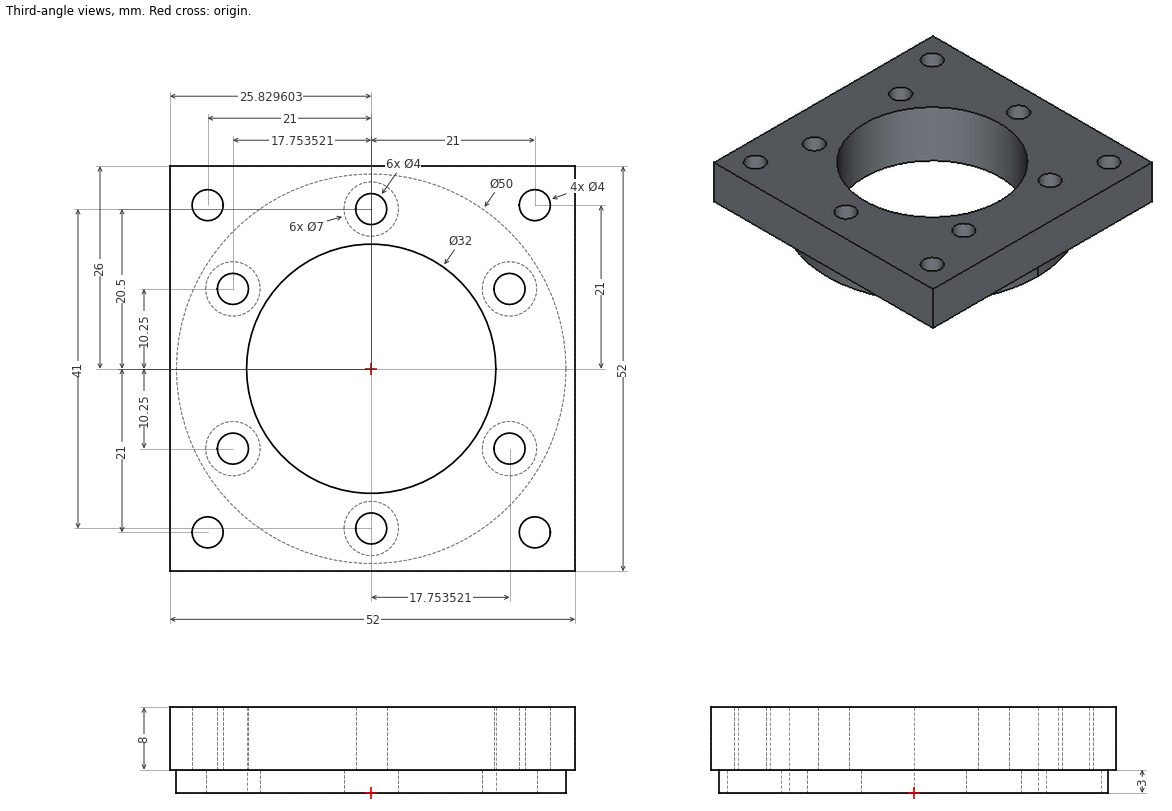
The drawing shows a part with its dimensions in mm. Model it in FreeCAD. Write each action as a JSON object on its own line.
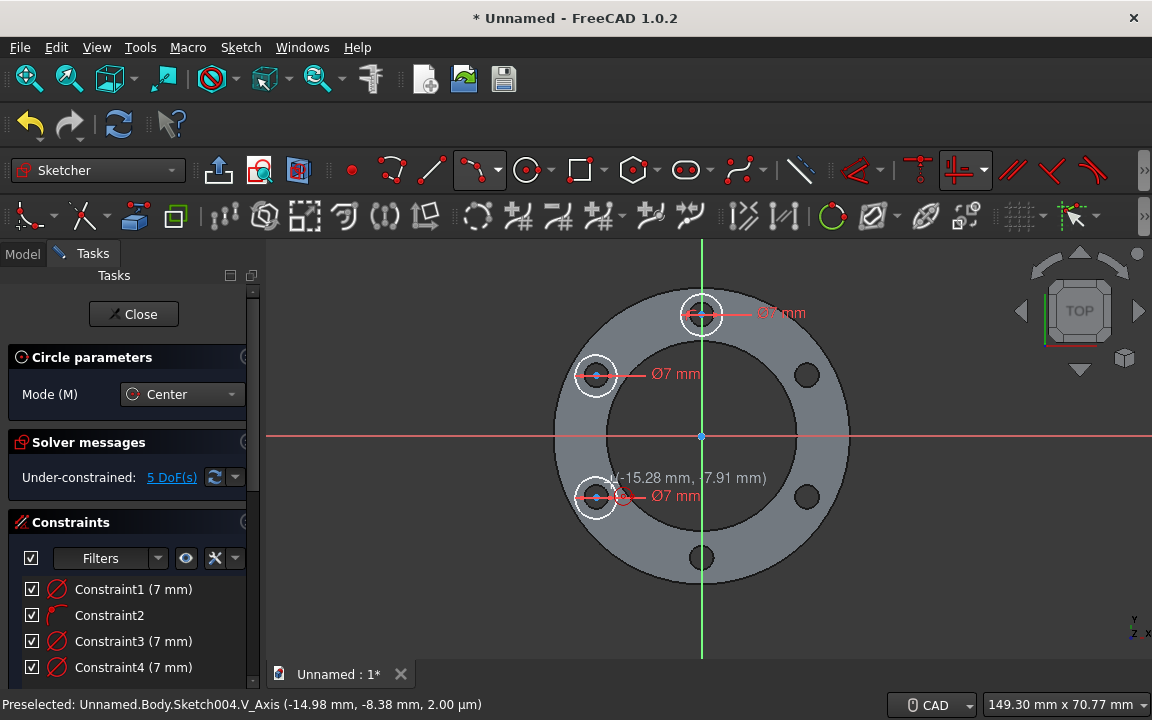
{"action": "left_click", "coordinate": [702, 558]}
{"action": "mouse_move", "coordinate": [716, 543]}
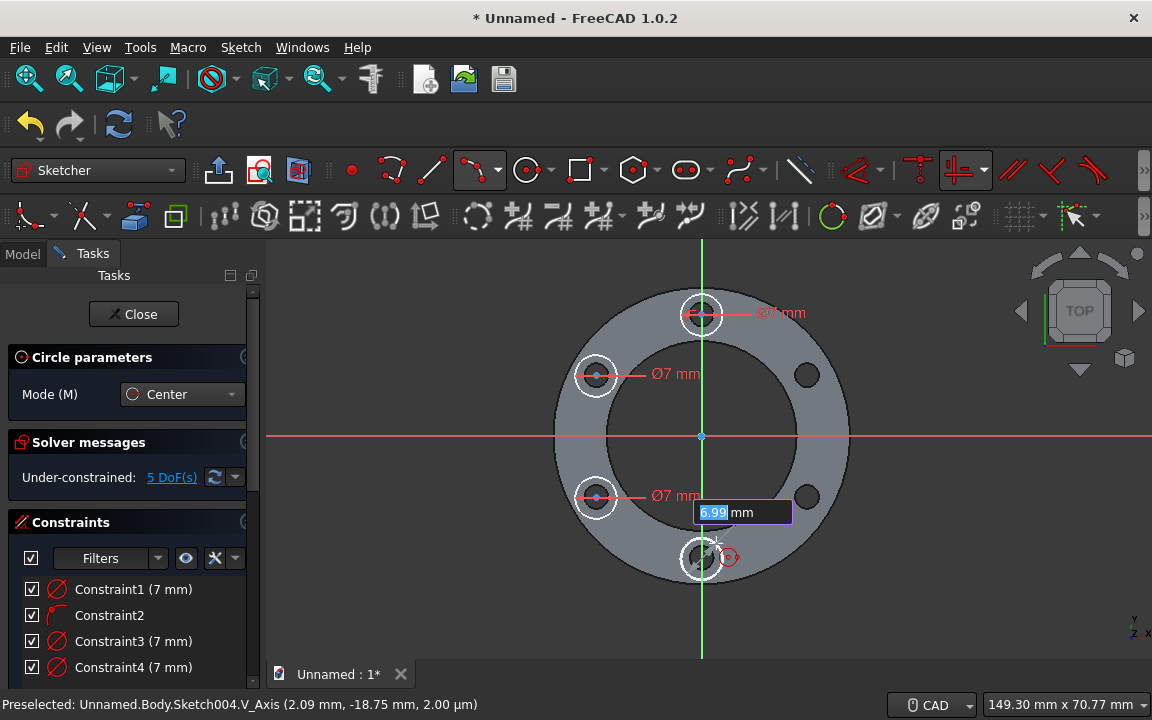
{"action": "type", "text": "7"}
{"action": "key", "text": "Return"}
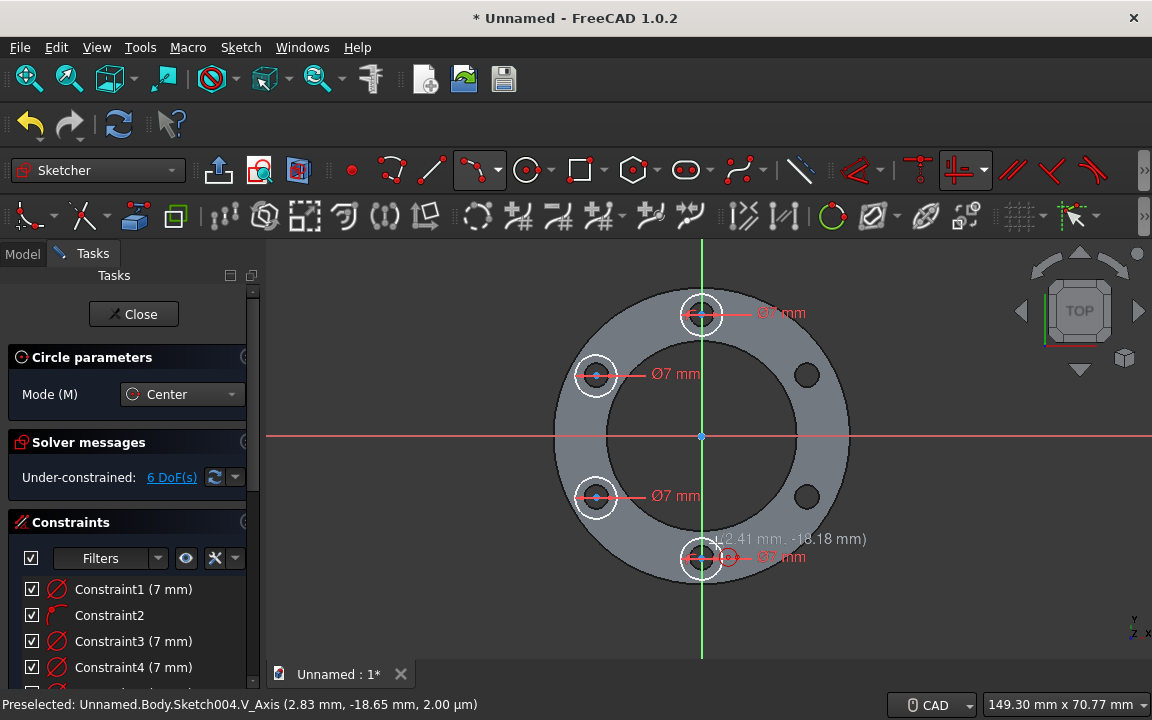
{"action": "left_click", "coordinate": [807, 497]}
{"action": "mouse_move", "coordinate": [822, 482]}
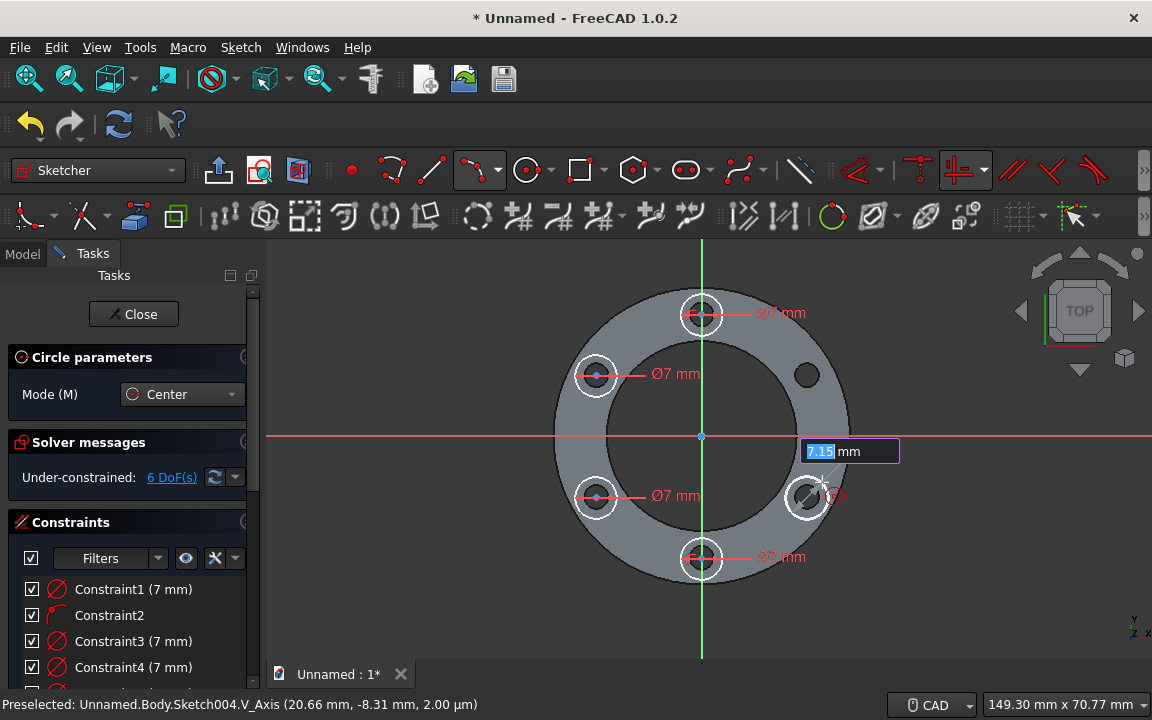
{"action": "type", "text": "7"}
{"action": "key", "text": "Return"}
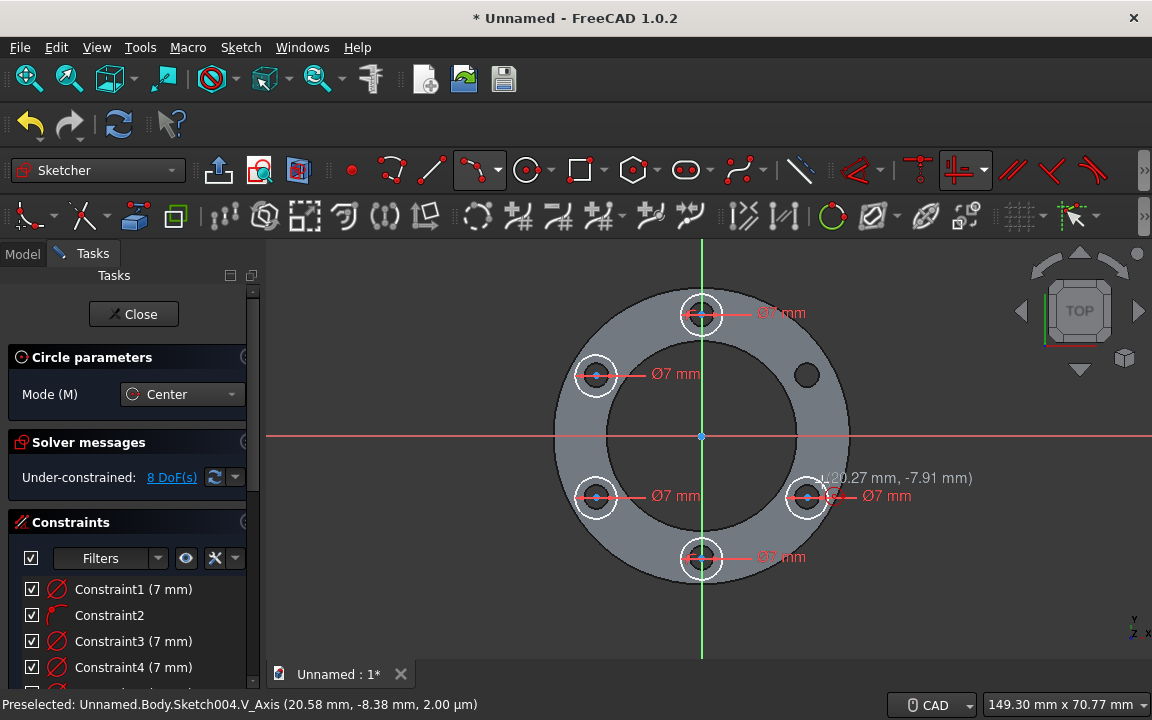
{"action": "left_click", "coordinate": [807, 375]}
{"action": "mouse_move", "coordinate": [822, 361]}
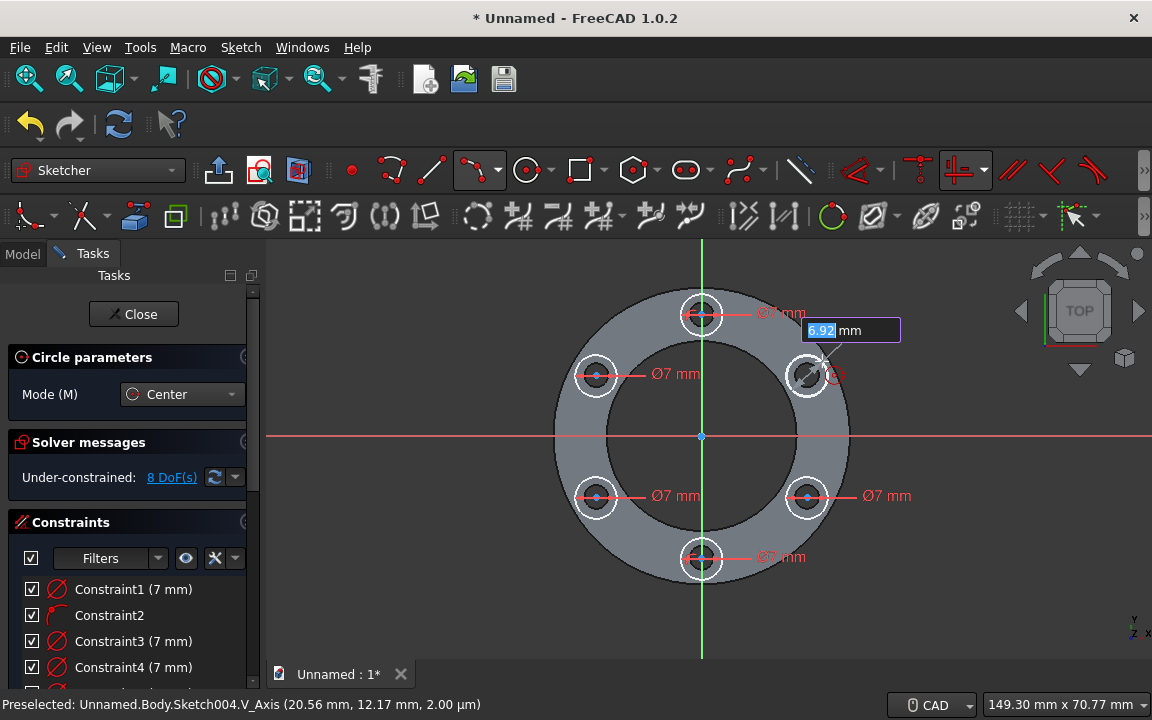
{"action": "type", "text": "7"}
{"action": "key", "text": "Return"}
{"action": "key", "text": "Escape"}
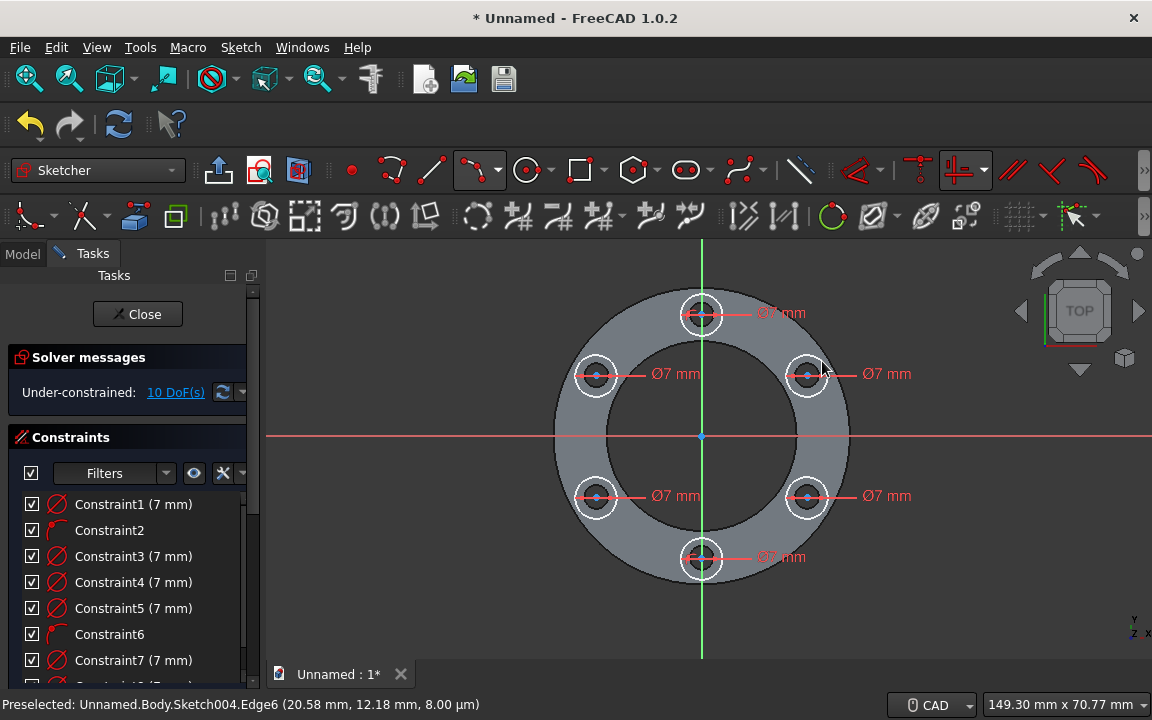
{"action": "left_click", "coordinate": [596, 376]}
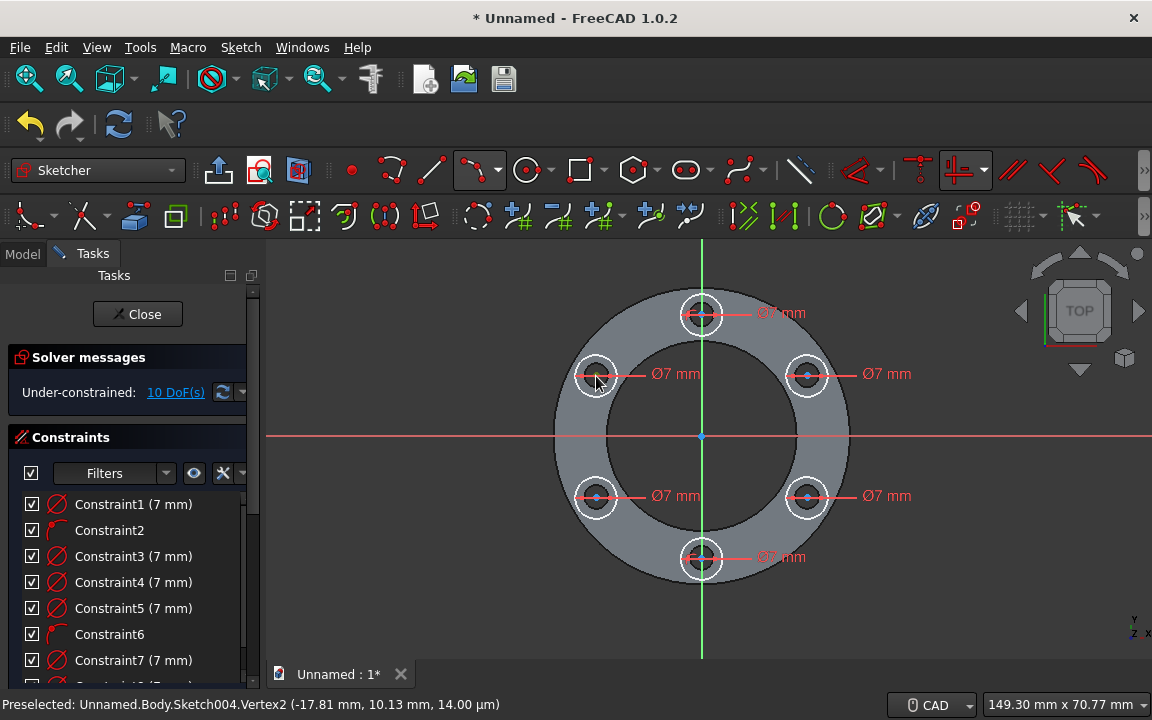
{"action": "left_click", "coordinate": [596, 498]}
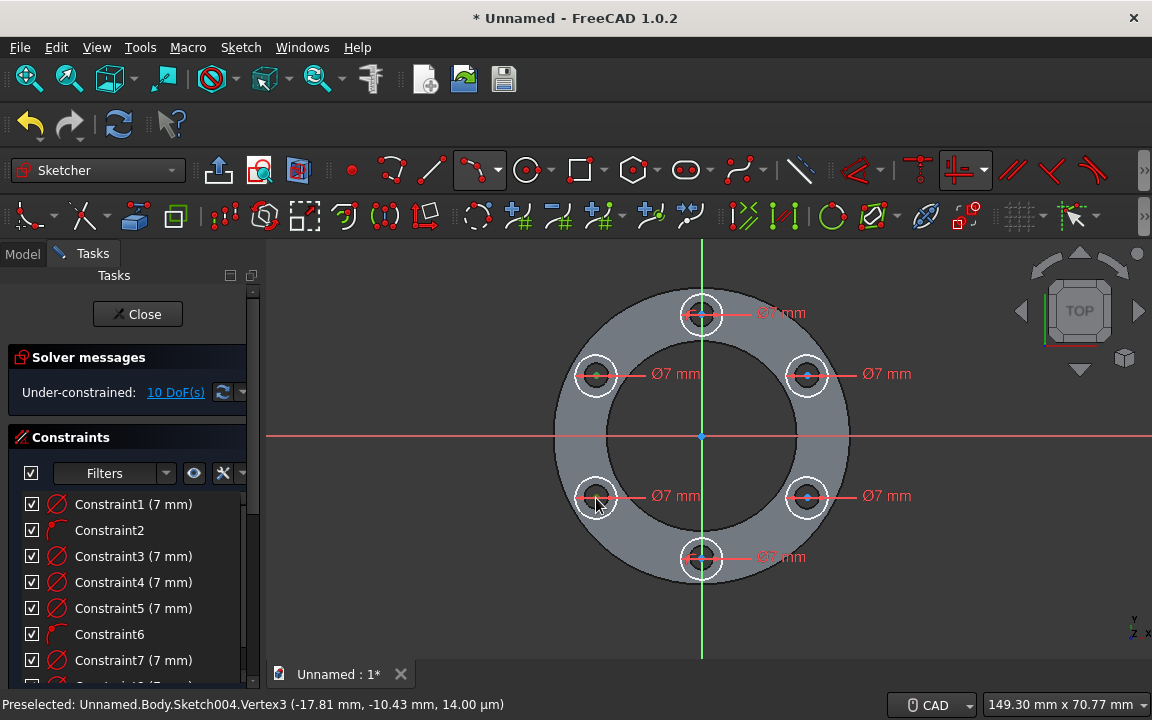
{"action": "key", "text": "v"}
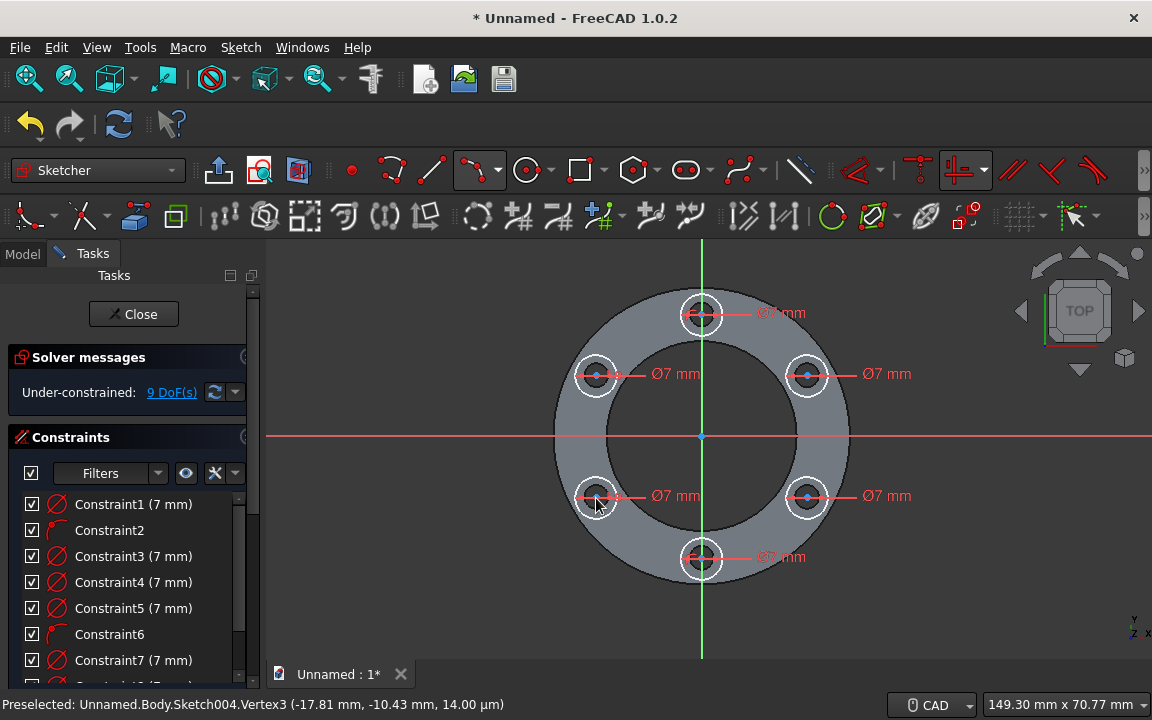
{"action": "left_click", "coordinate": [596, 498]}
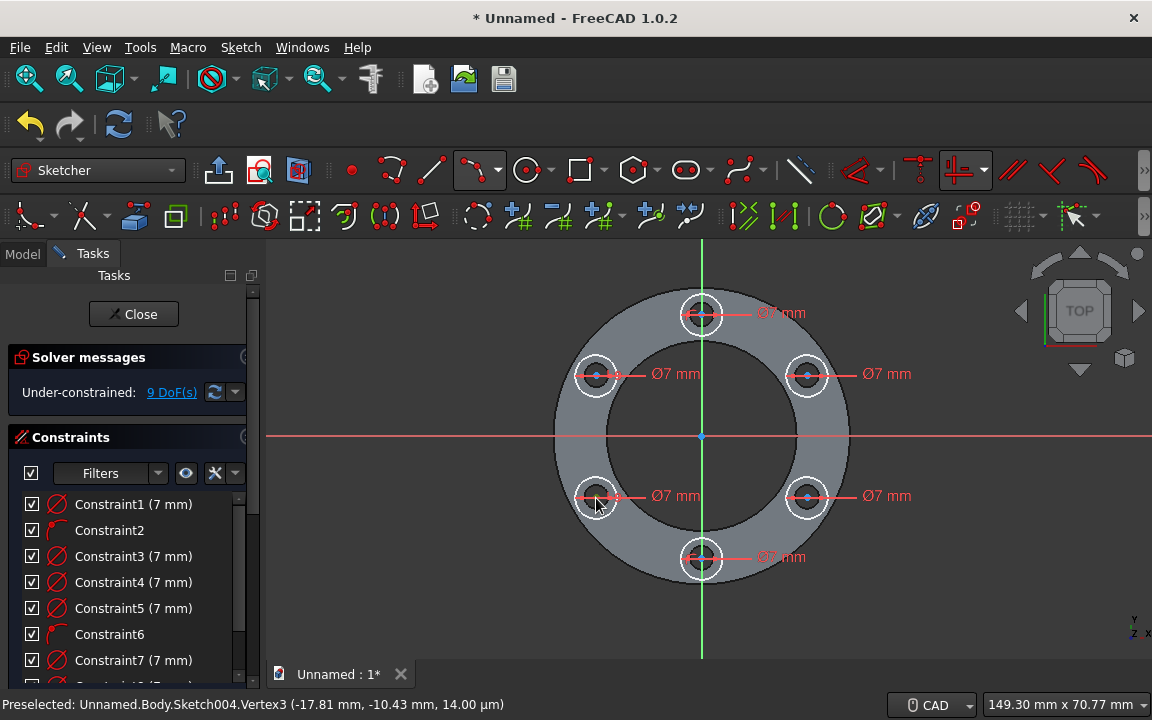
{"action": "left_click", "coordinate": [807, 498]}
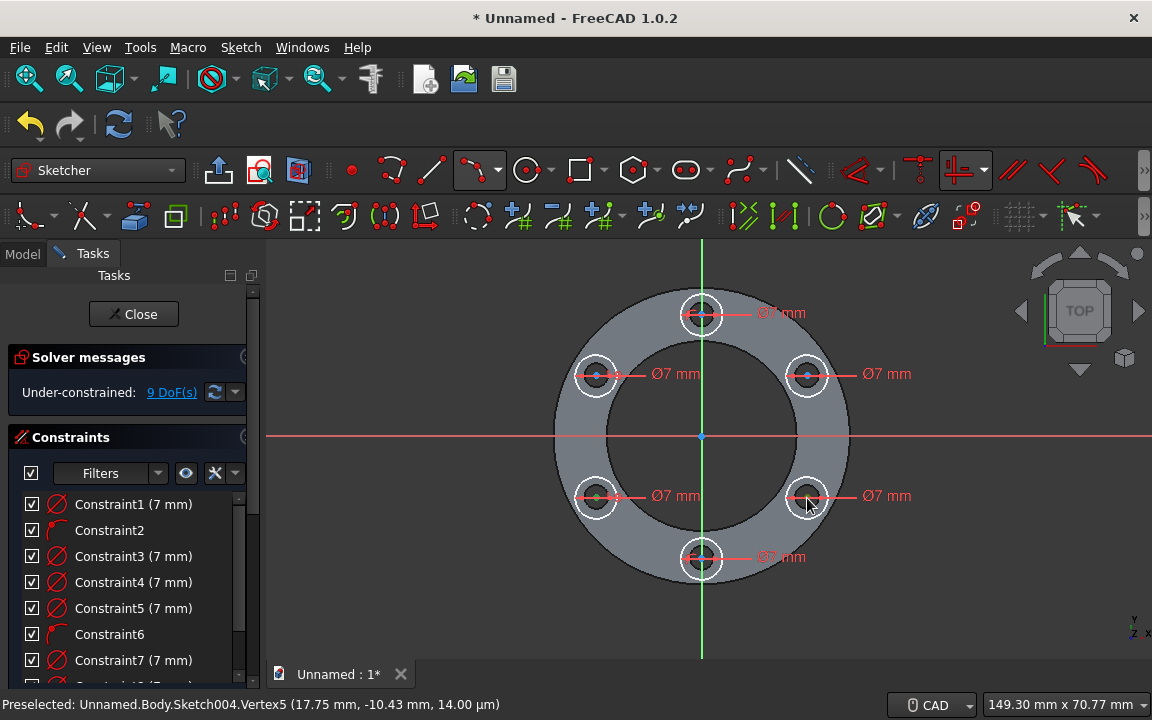
{"action": "key", "text": "h"}